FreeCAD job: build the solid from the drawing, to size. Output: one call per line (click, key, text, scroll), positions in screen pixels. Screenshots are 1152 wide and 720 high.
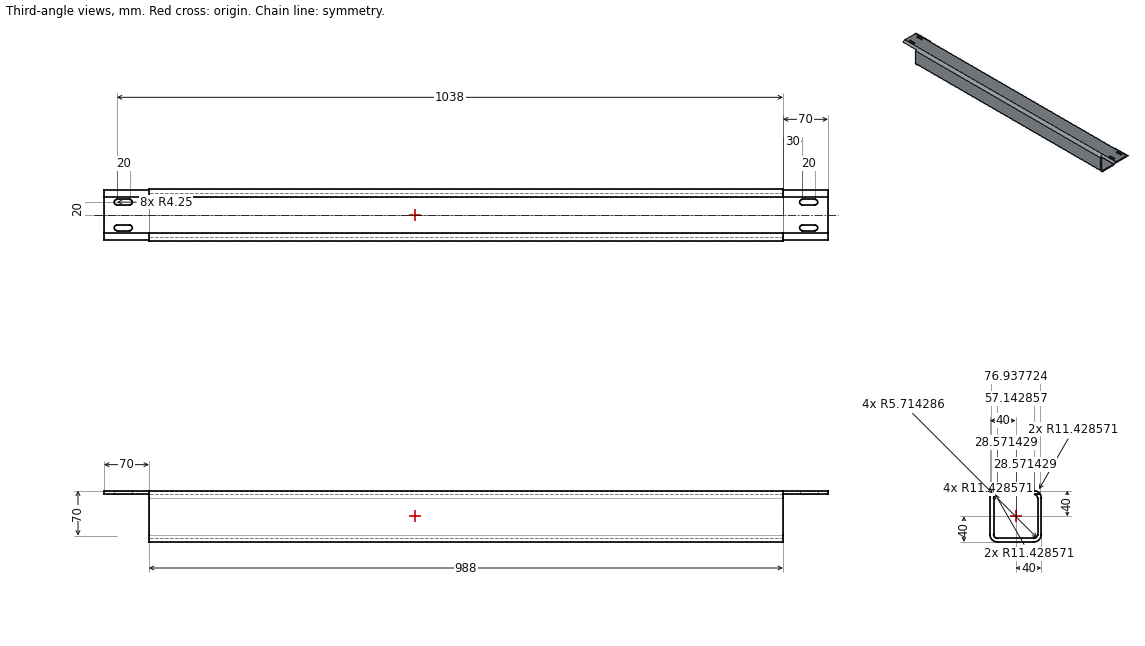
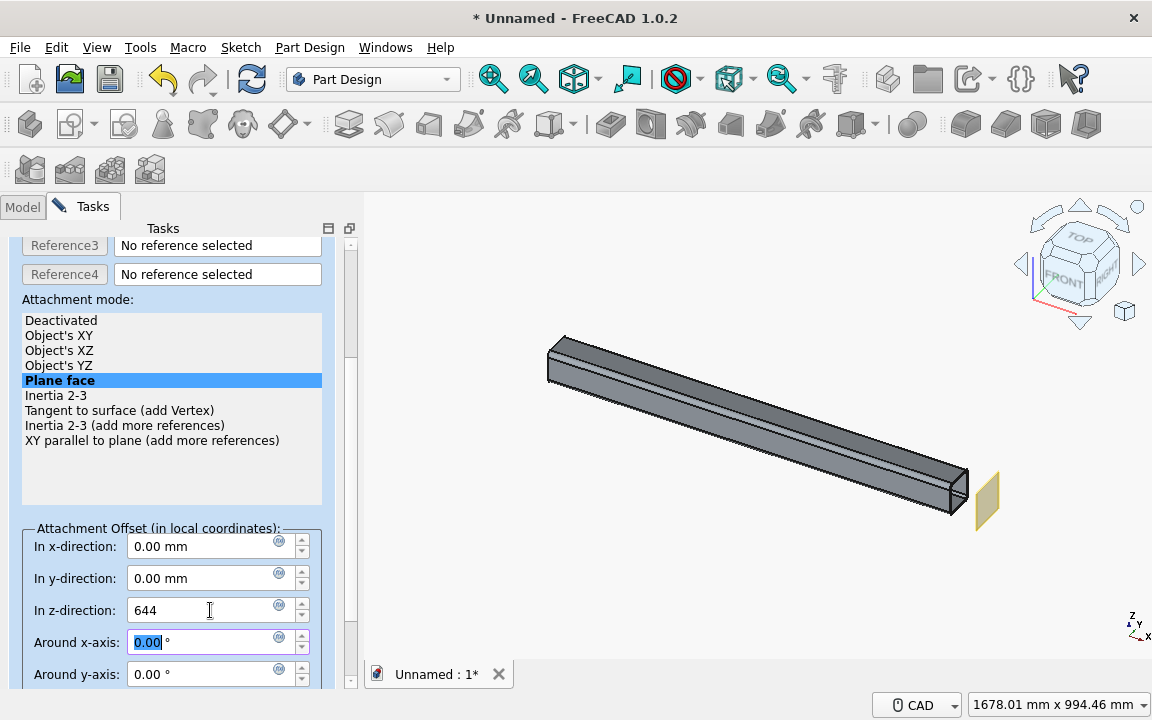
scroll(351, 463, up, 4)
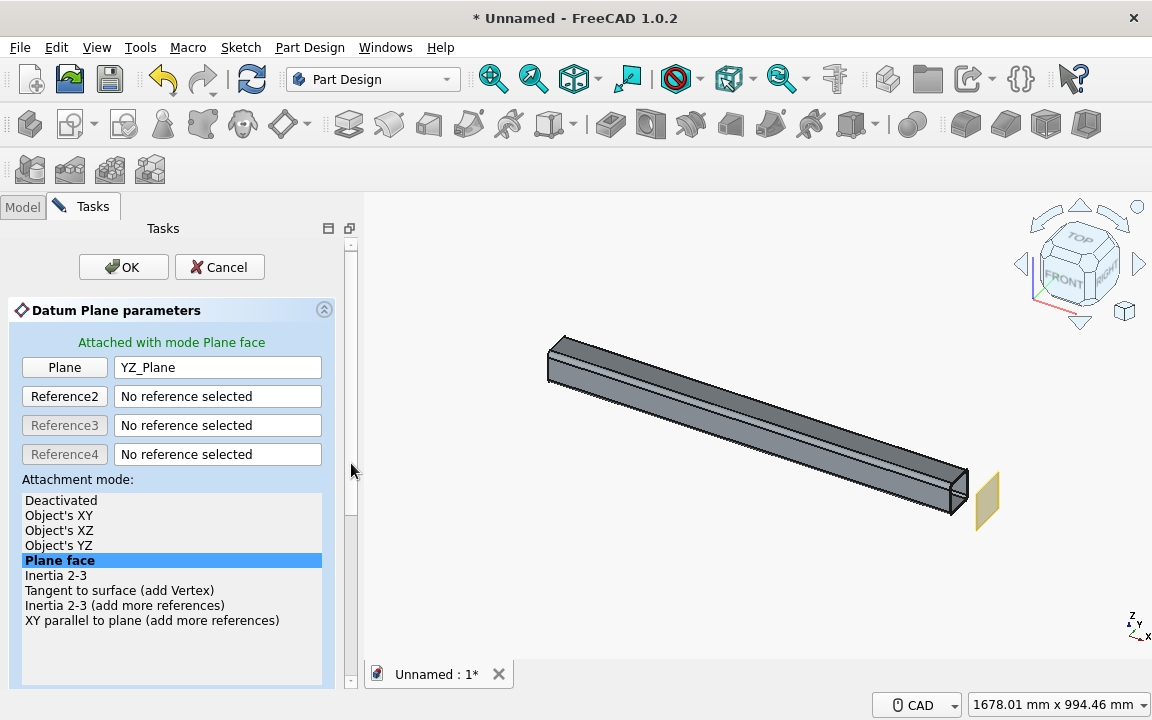
click(124, 267)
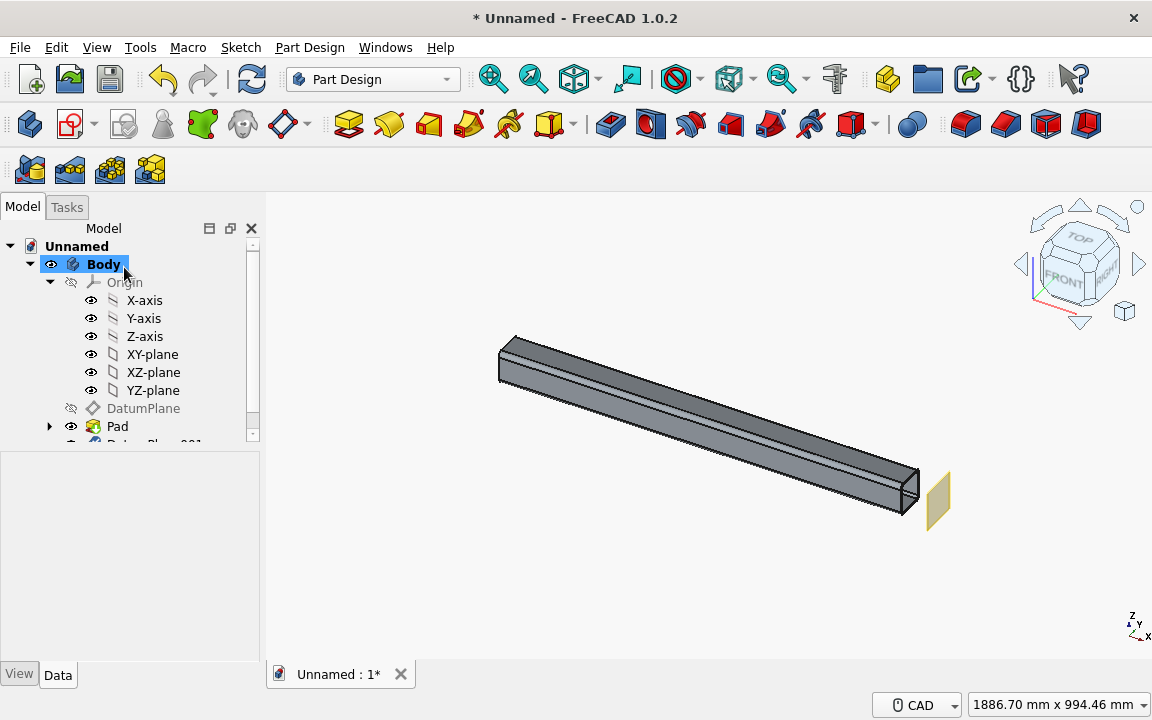
scroll(100, 332, down, 3)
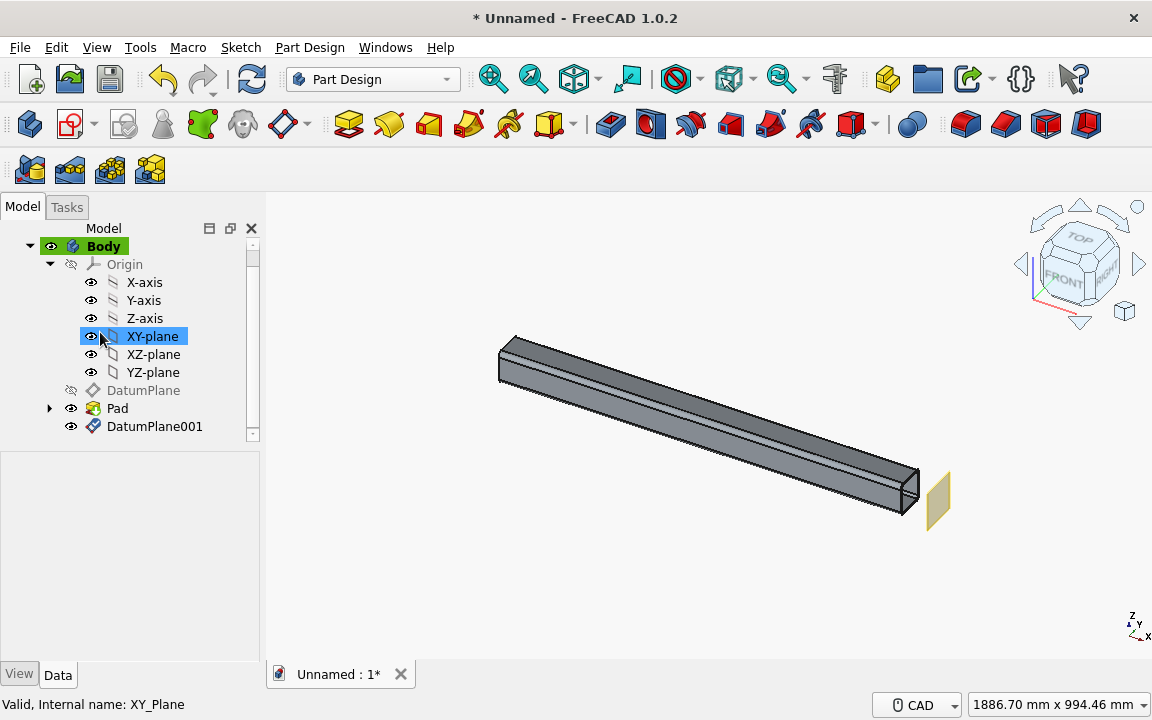
click(116, 426)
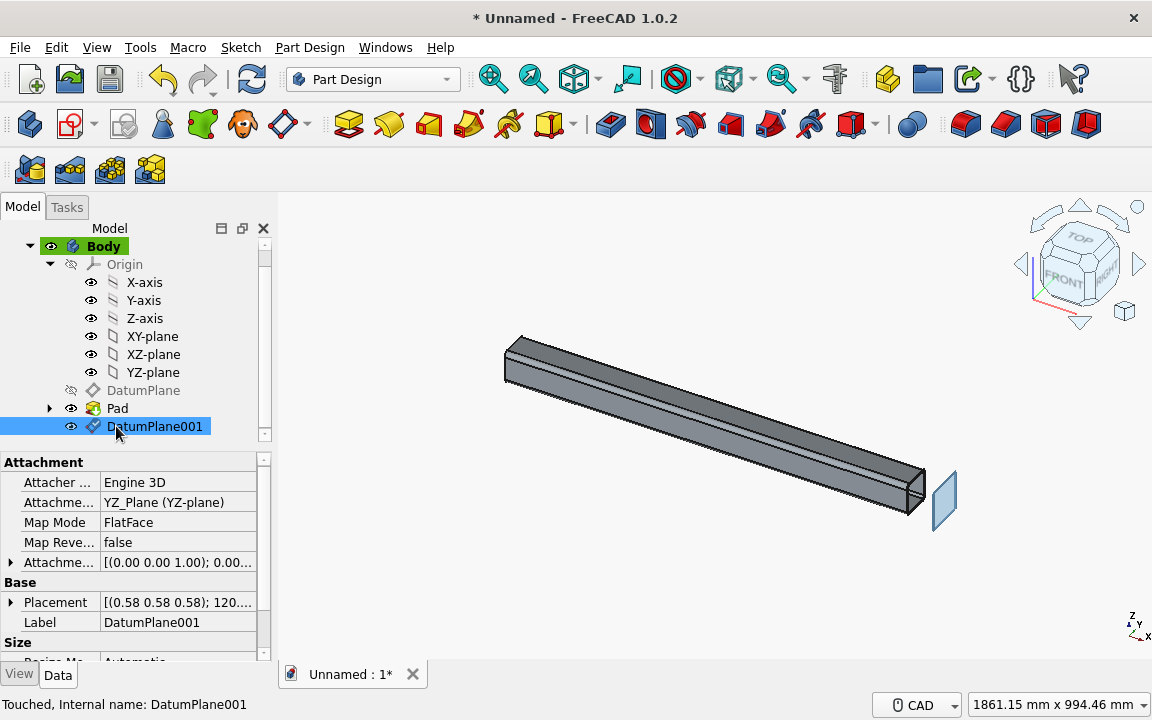
click(70, 124)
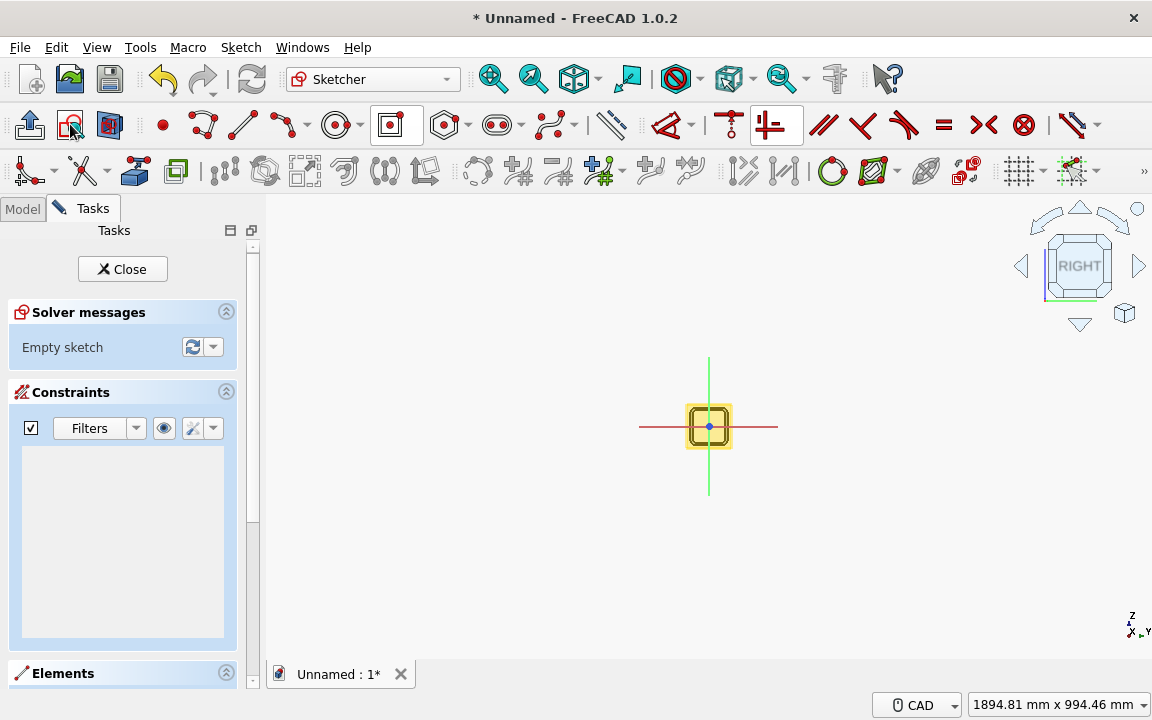
scroll(714, 416, up, 13)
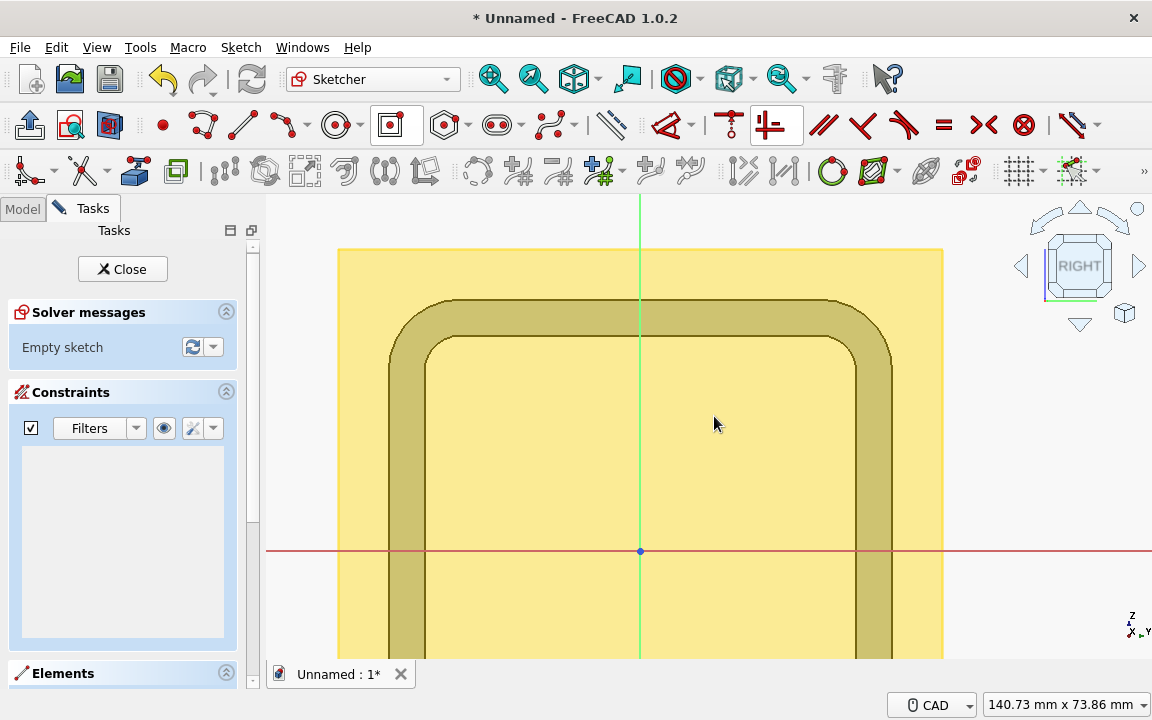
key(g)
key(l)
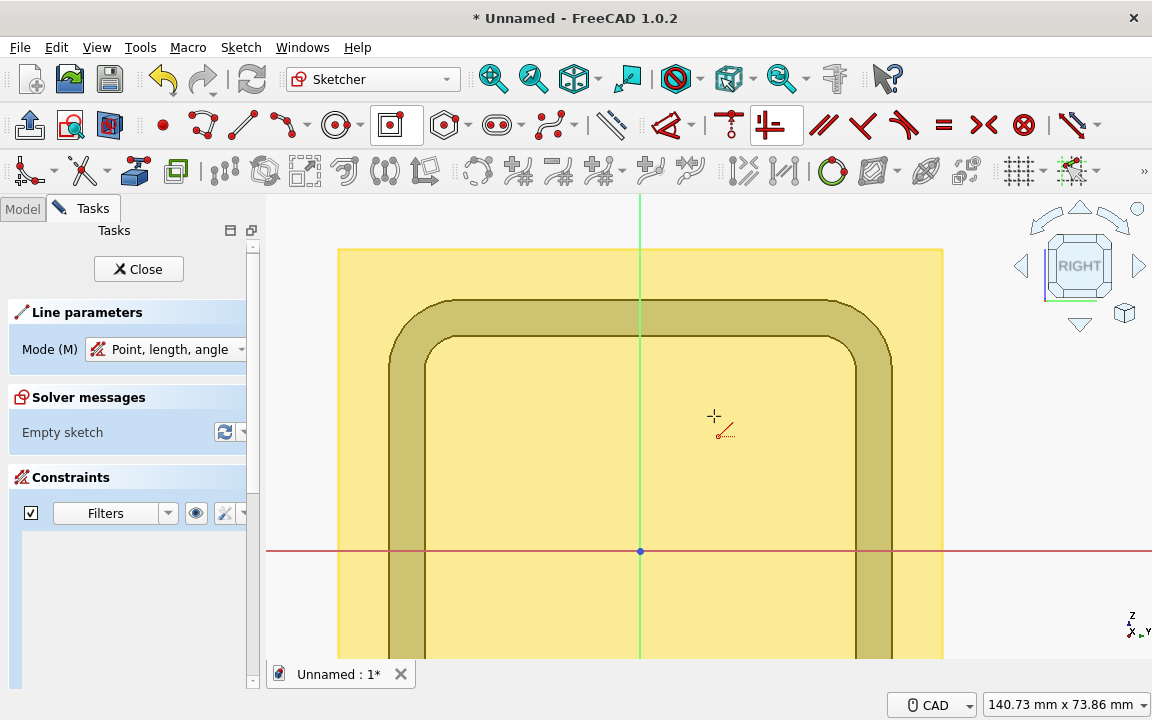
click(820, 300)
click(460, 300)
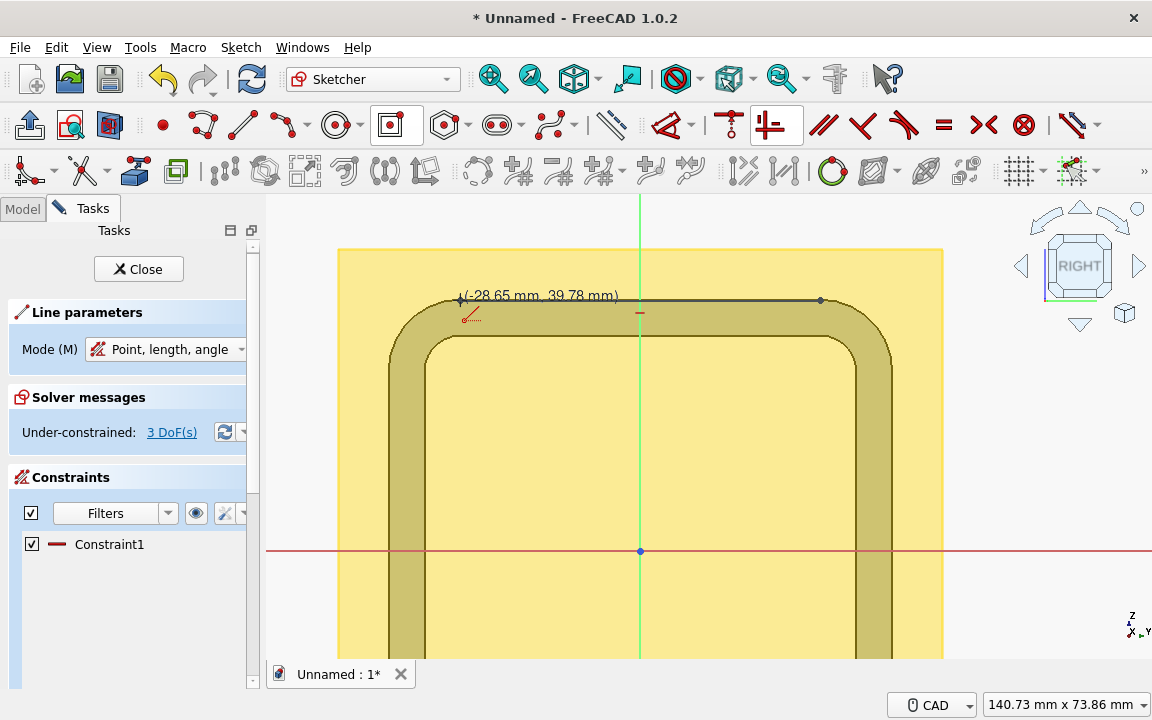
click(398, 336)
click(883, 336)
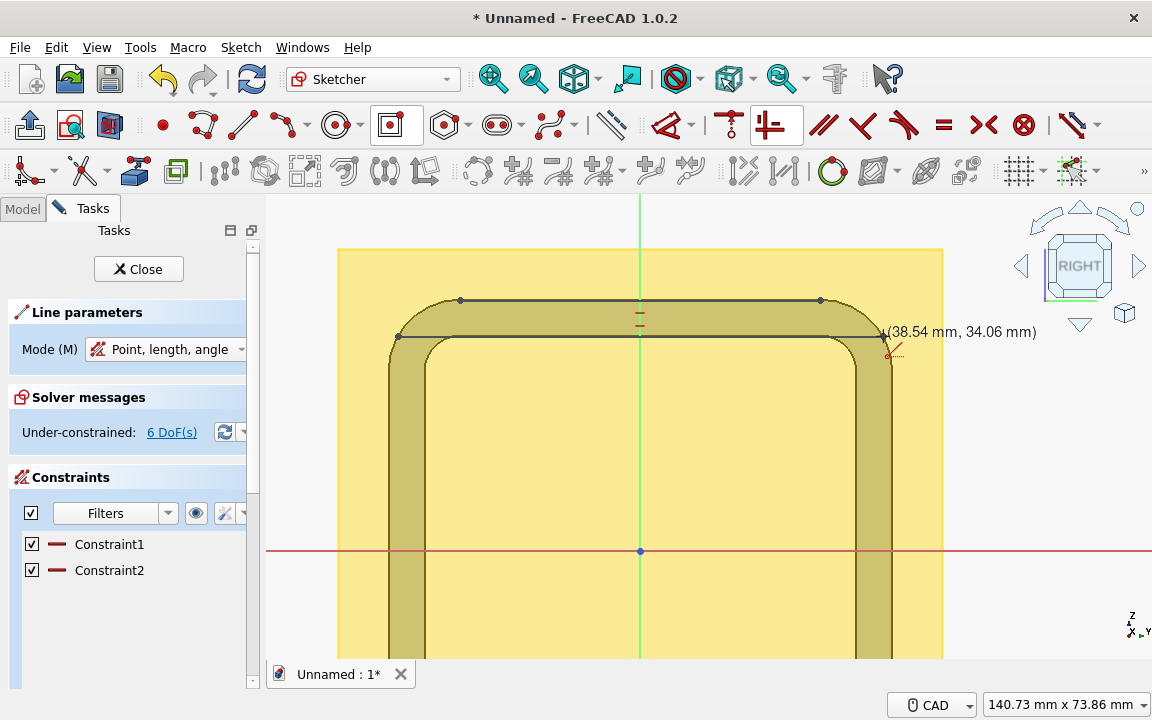
click(284, 126)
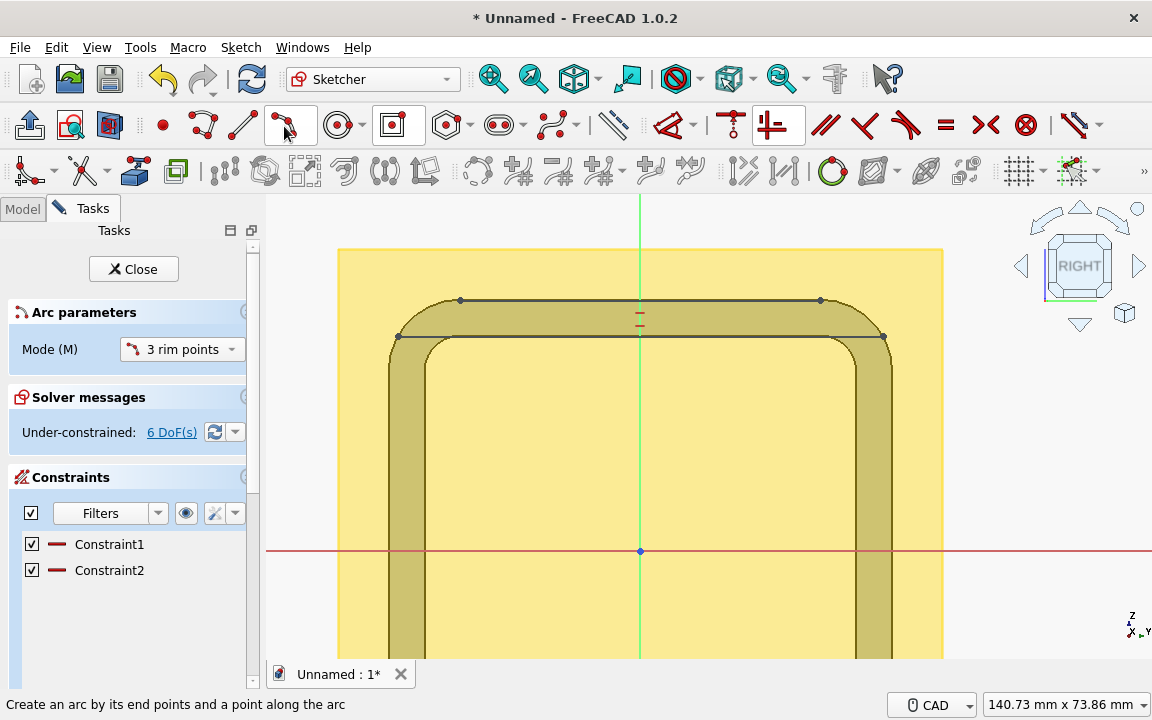
click(460, 301)
click(398, 337)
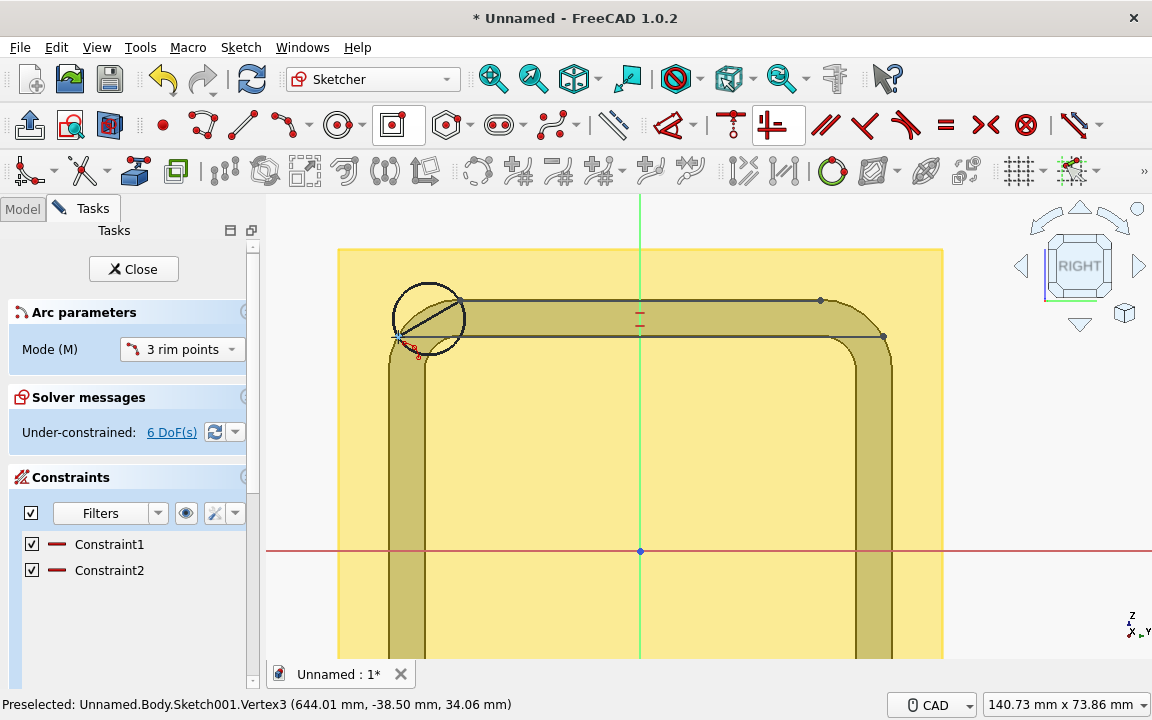
scroll(425, 309, up, 3)